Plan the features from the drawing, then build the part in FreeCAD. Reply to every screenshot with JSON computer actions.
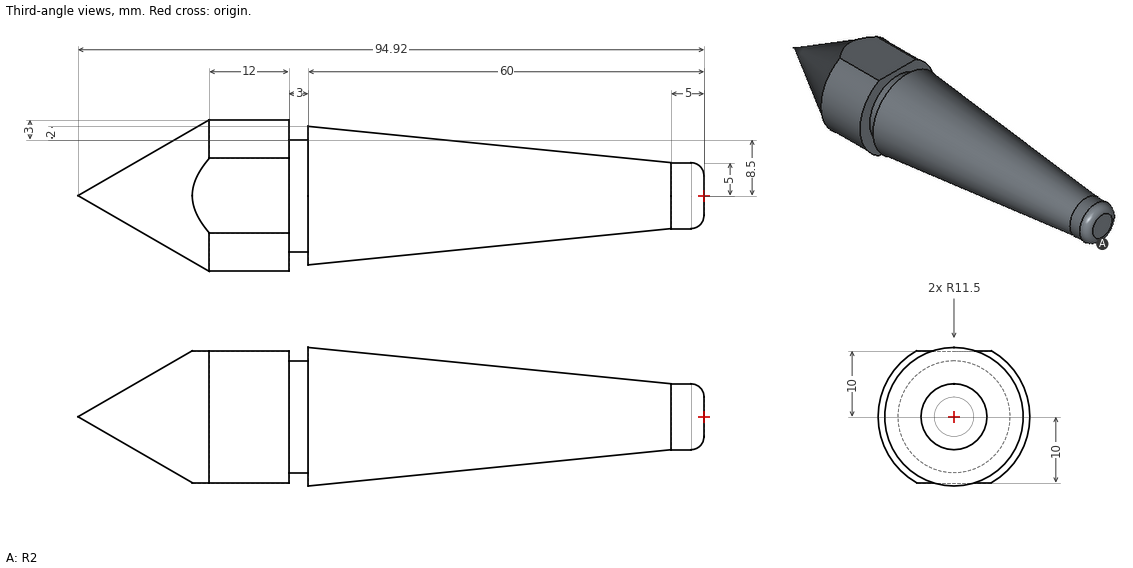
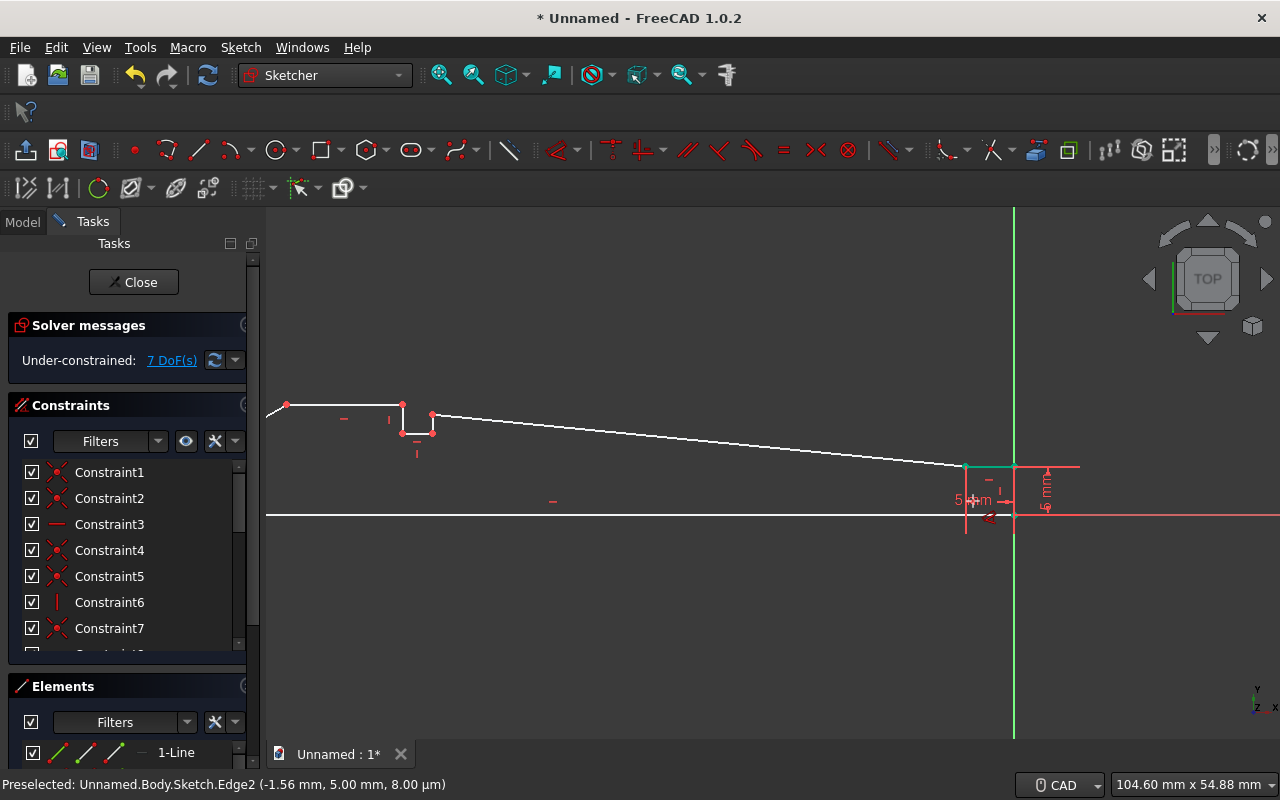
{"action": "scroll", "coordinate": [433, 424], "scroll_direction": "up", "scroll_amount": 4}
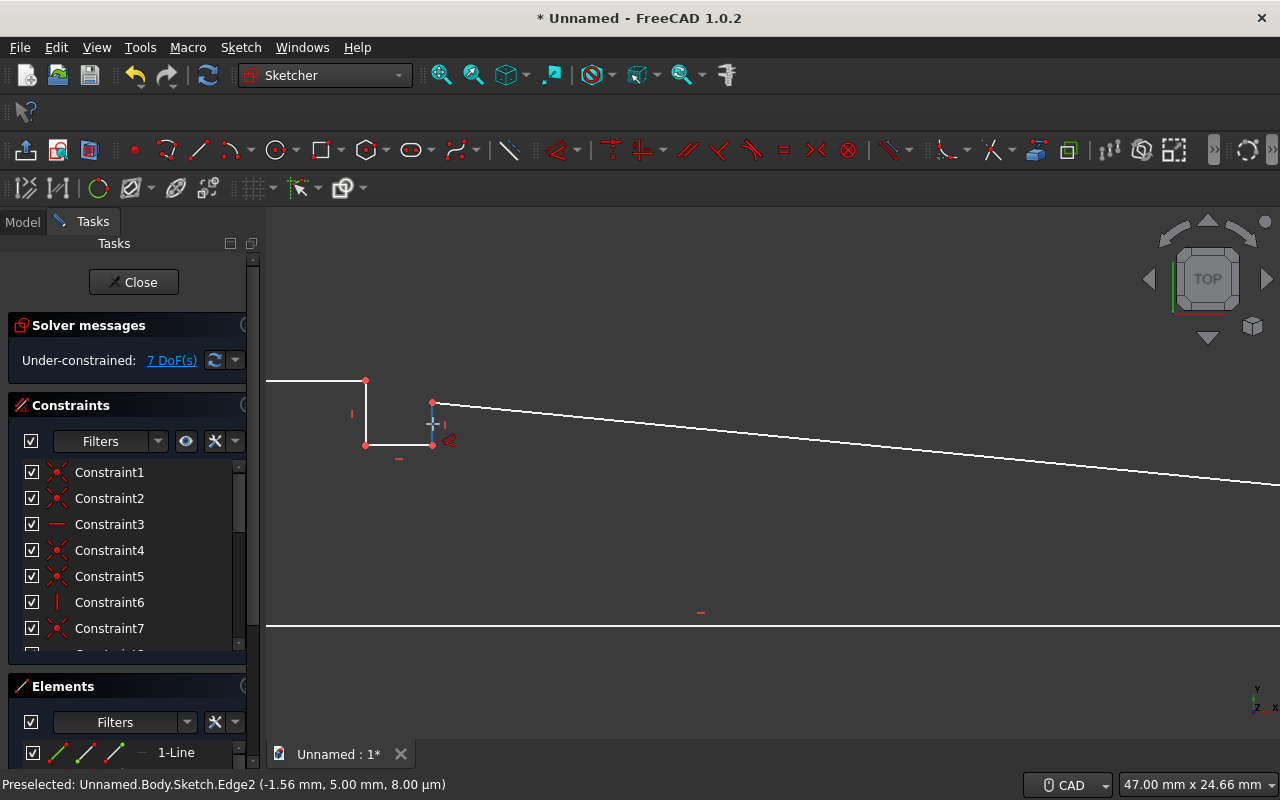
{"action": "left_click", "coordinate": [432, 424]}
{"action": "left_click", "coordinate": [398, 424]}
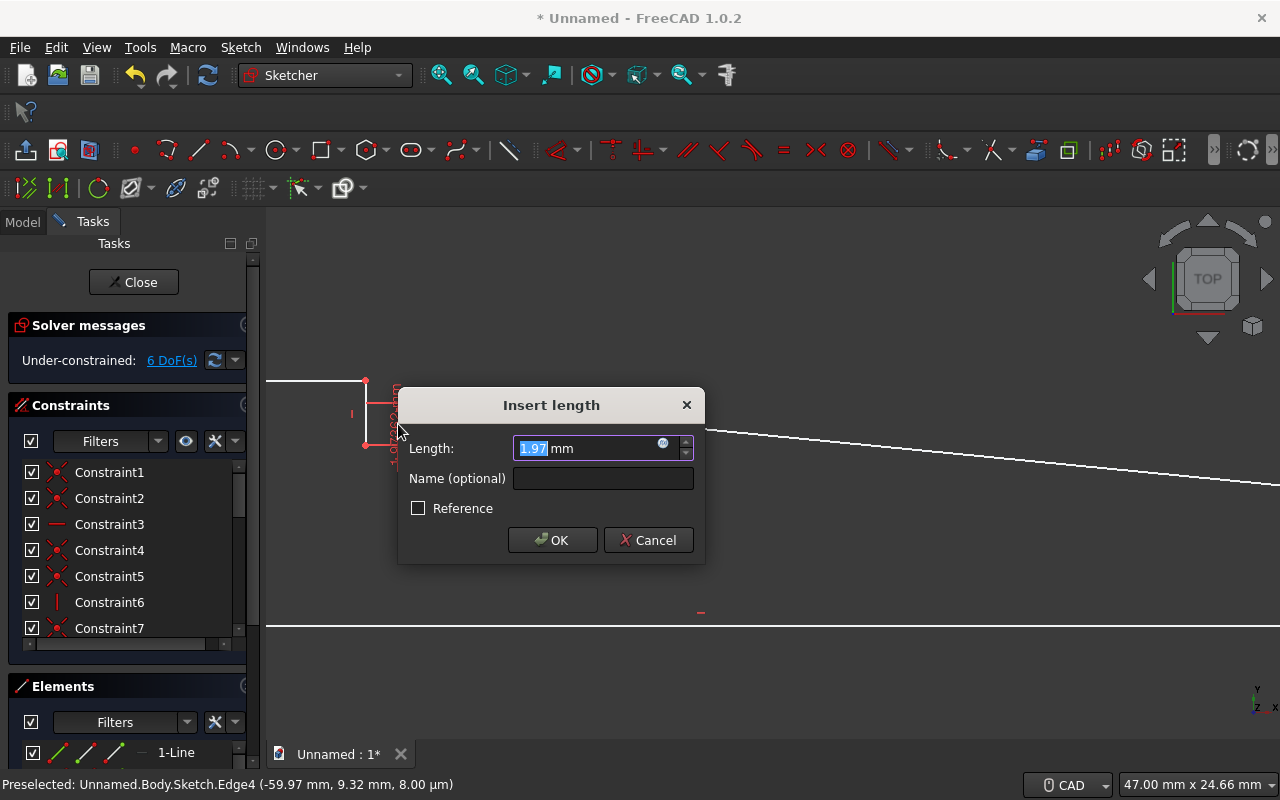
{"action": "type", "text": "2"}
{"action": "key", "text": "Return"}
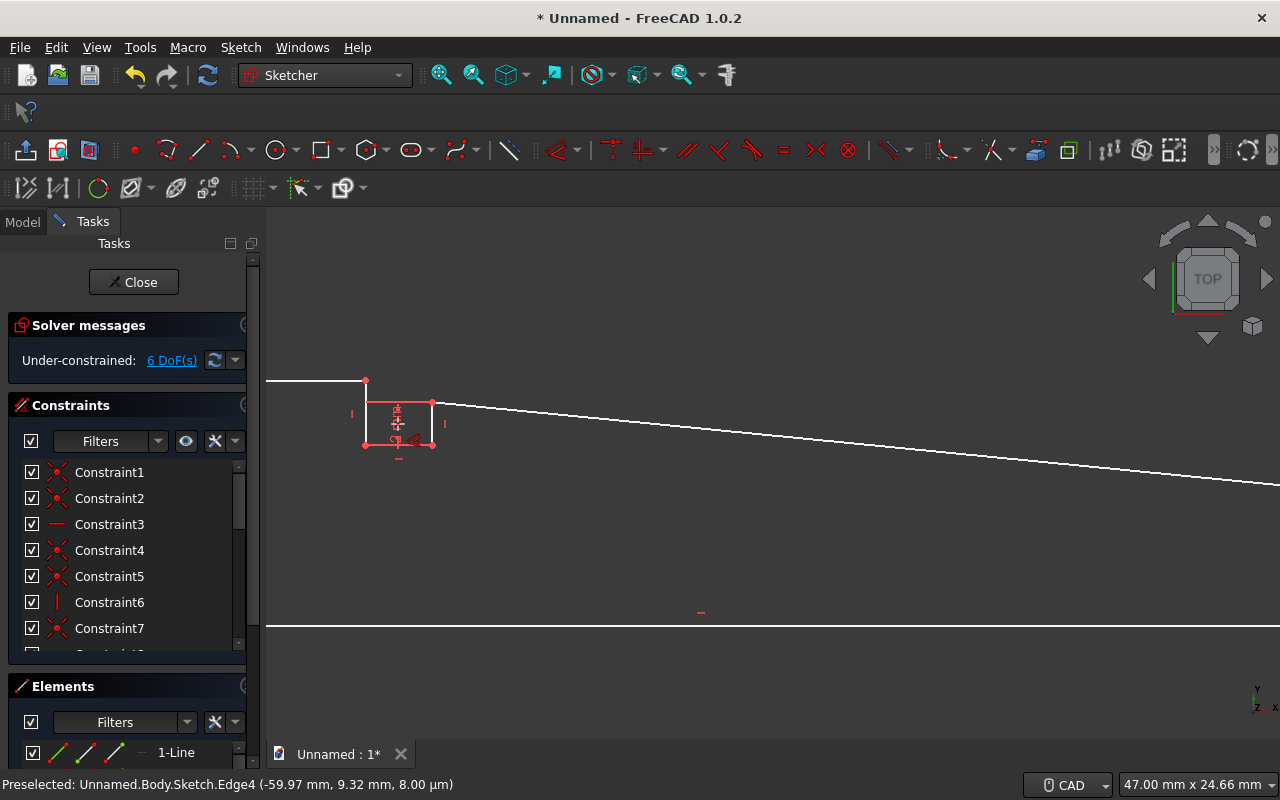
{"action": "left_click", "coordinate": [412, 445]}
{"action": "left_click", "coordinate": [399, 479]}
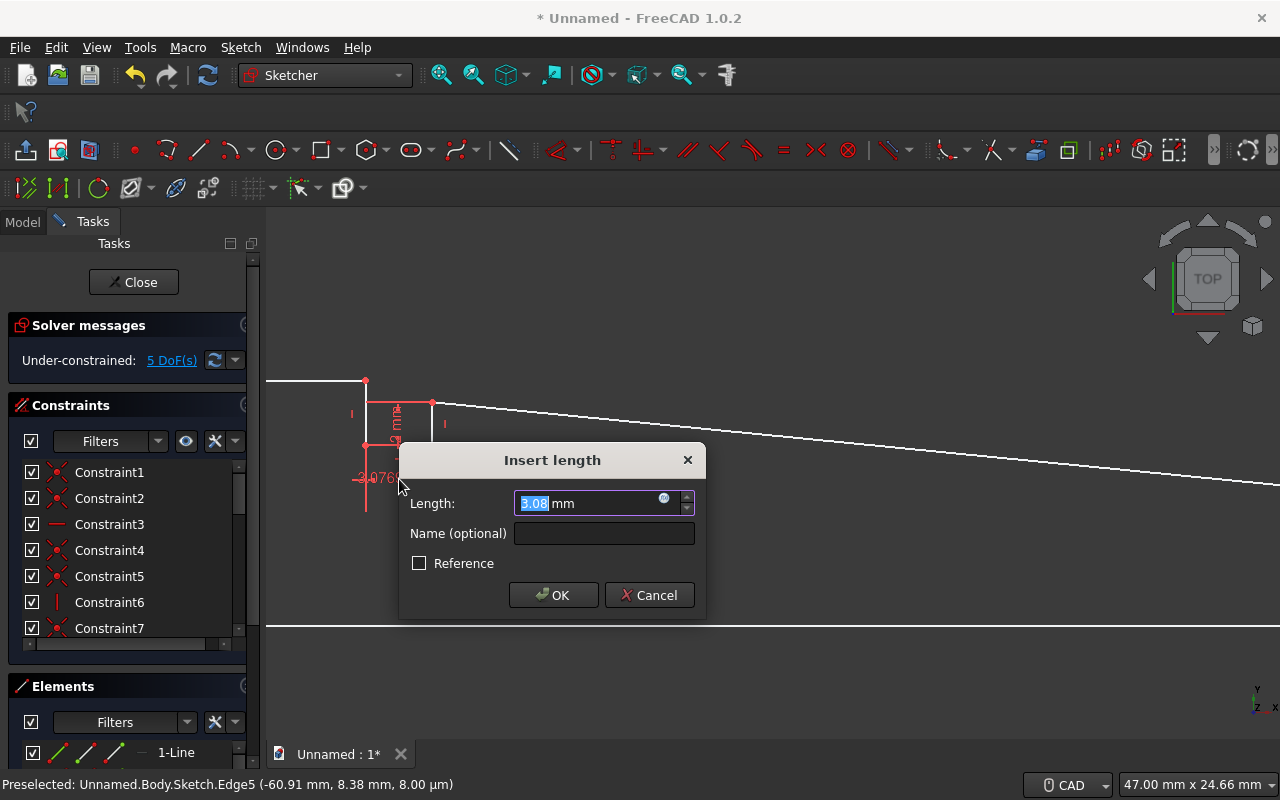
{"action": "type", "text": "3"}
{"action": "key", "text": "Return"}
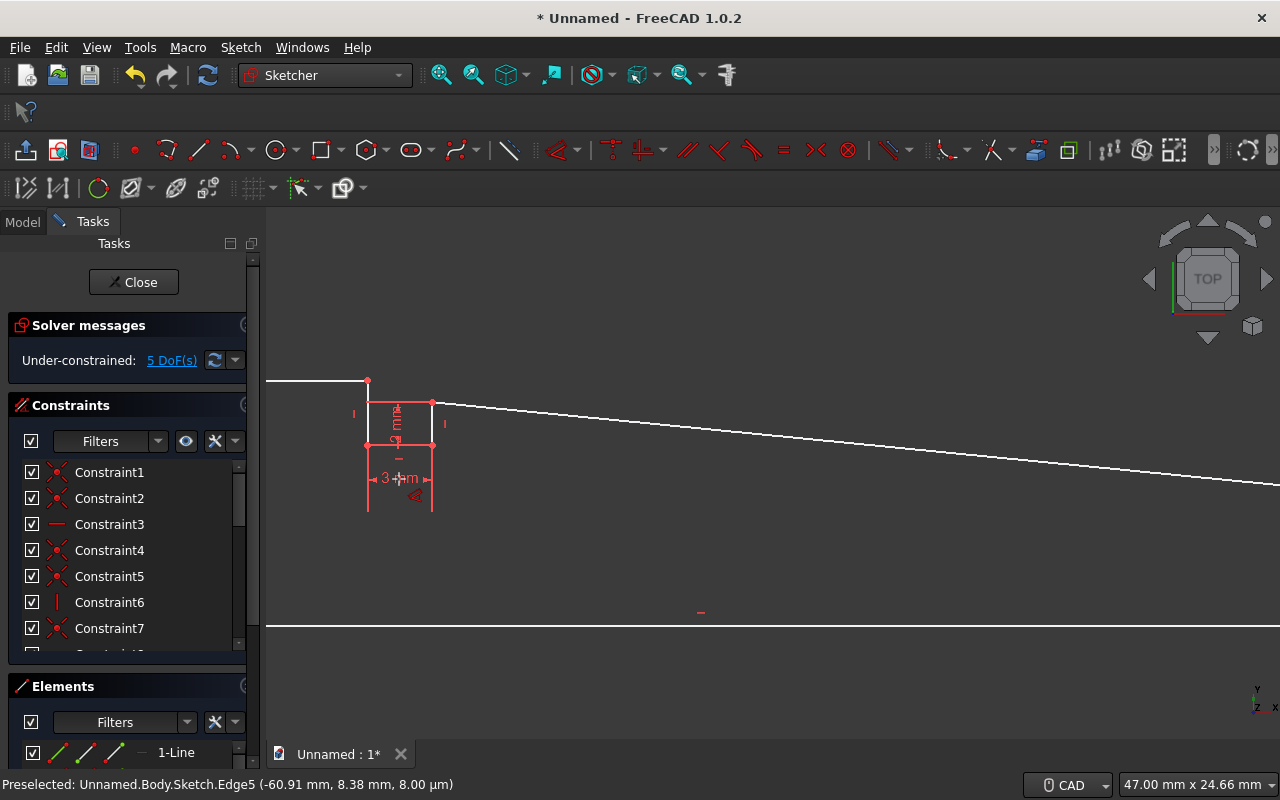
{"action": "left_click", "coordinate": [368, 426]}
{"action": "left_click", "coordinate": [334, 398]}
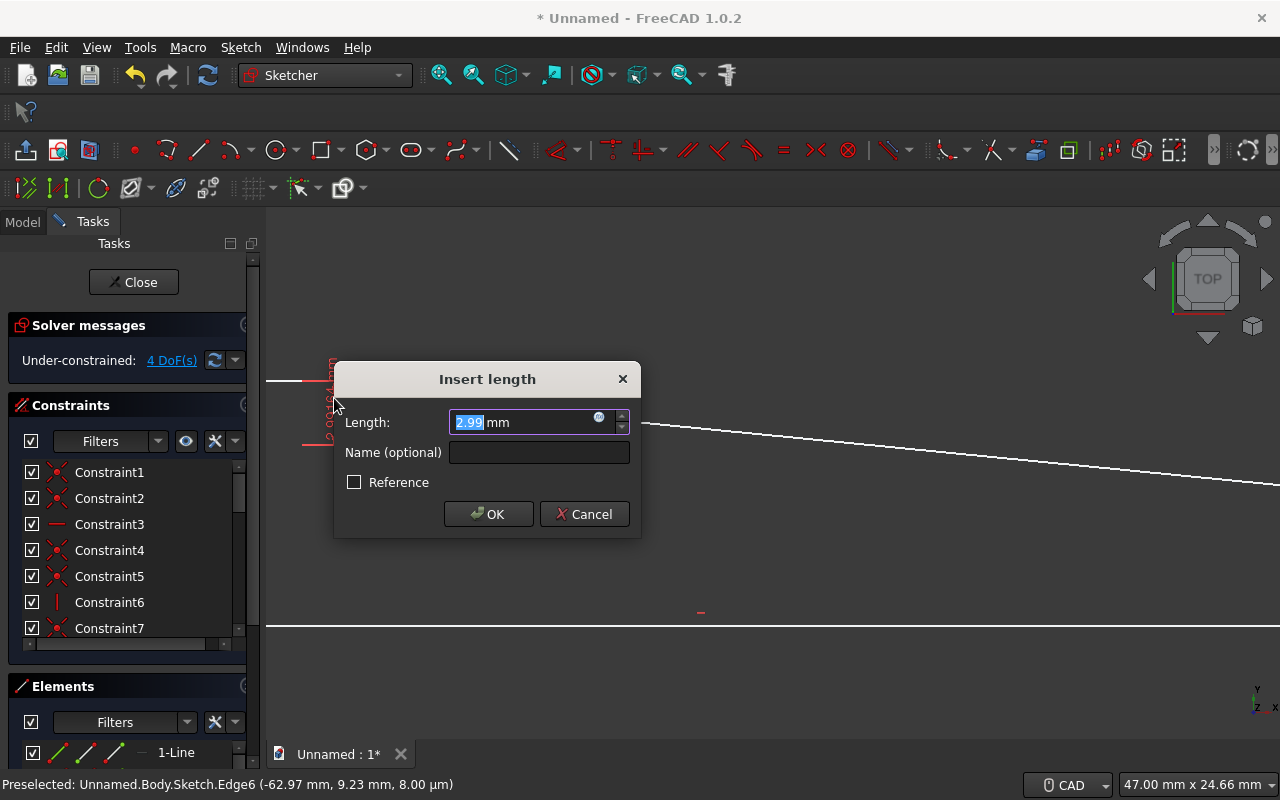
{"action": "type", "text": "3"}
{"action": "key", "text": "Return"}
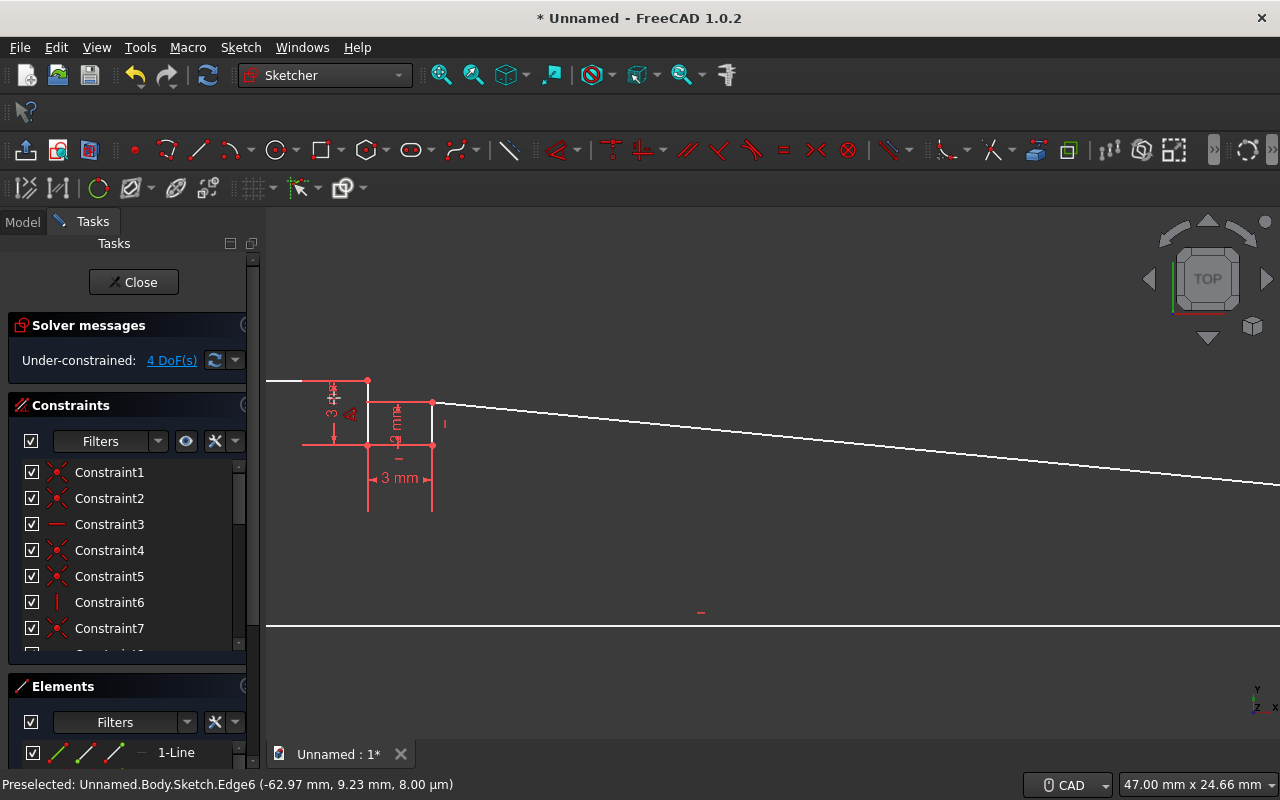
{"action": "left_click", "coordinate": [316, 381]}
{"action": "left_click", "coordinate": [331, 347]}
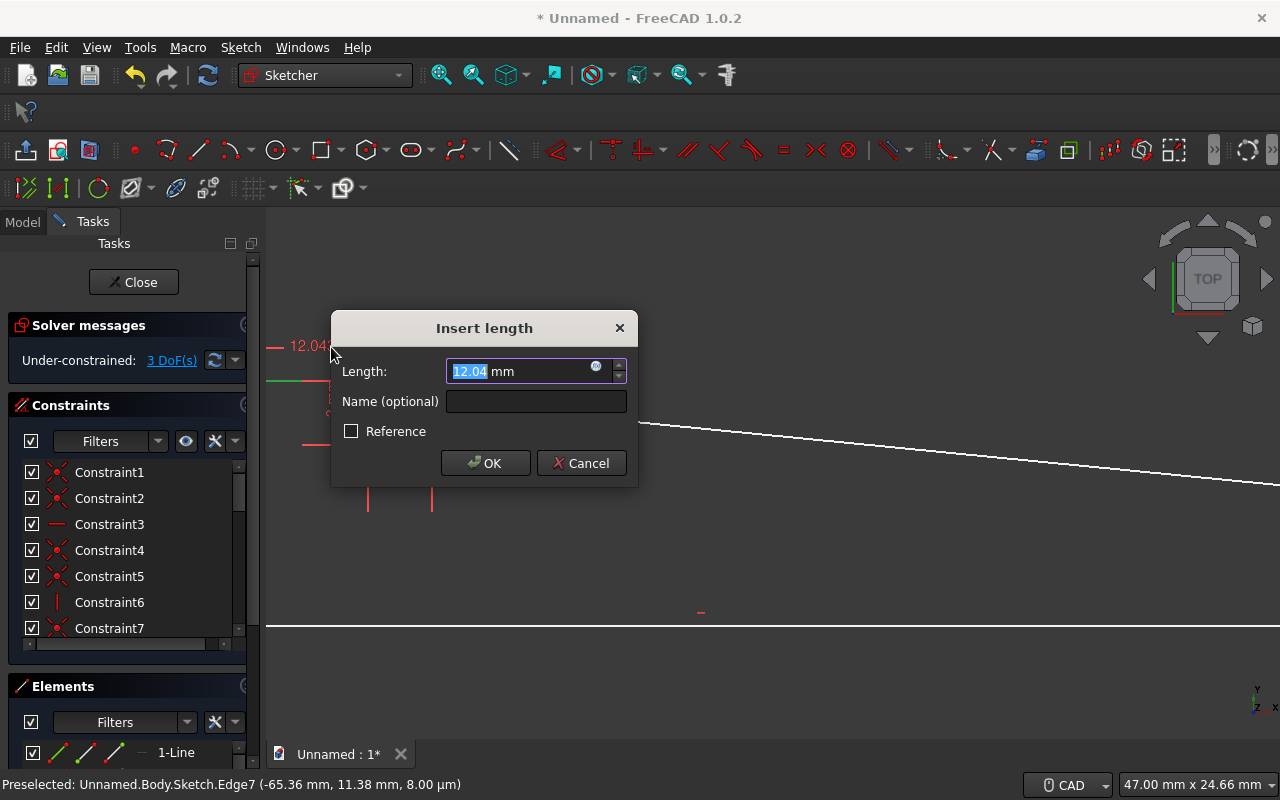
{"action": "type", "text": "12"}
{"action": "key", "text": "Return"}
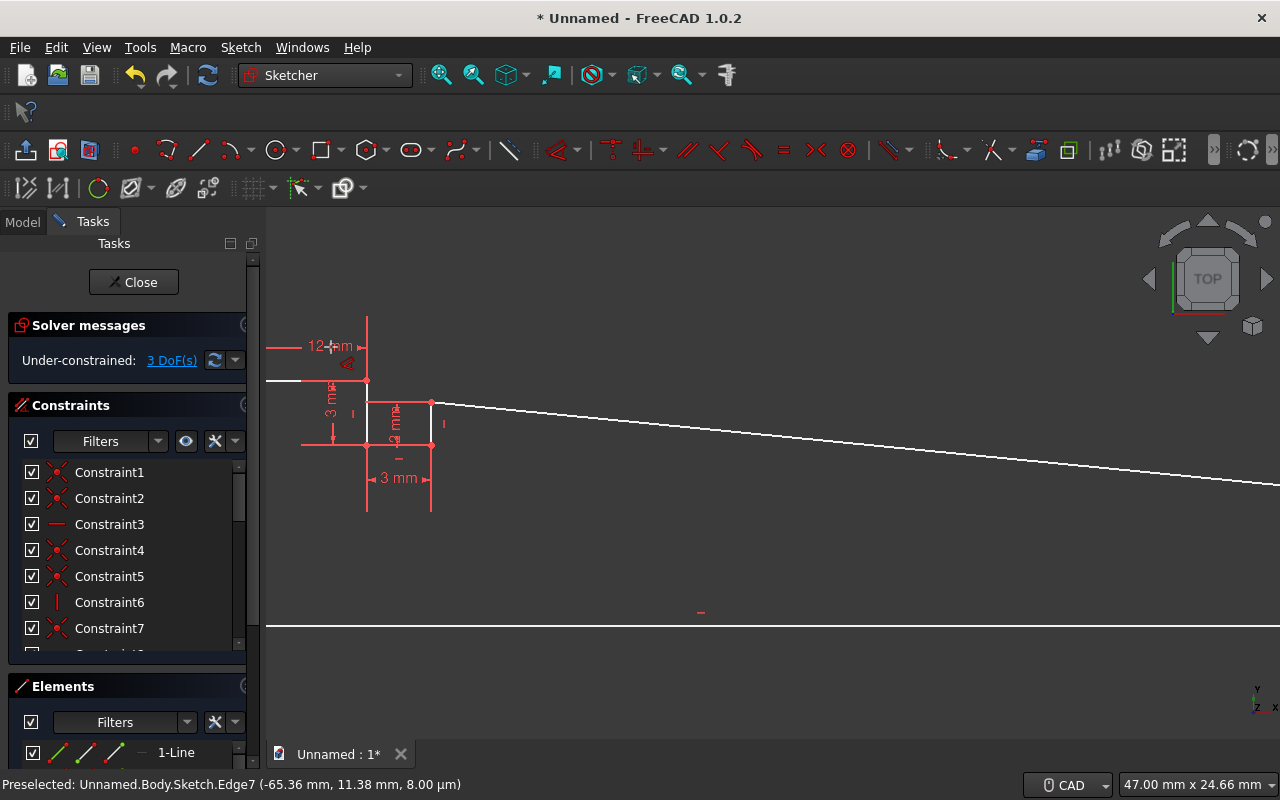
{"action": "left_click", "coordinate": [431, 402]}
{"action": "left_click", "coordinate": [773, 660]}